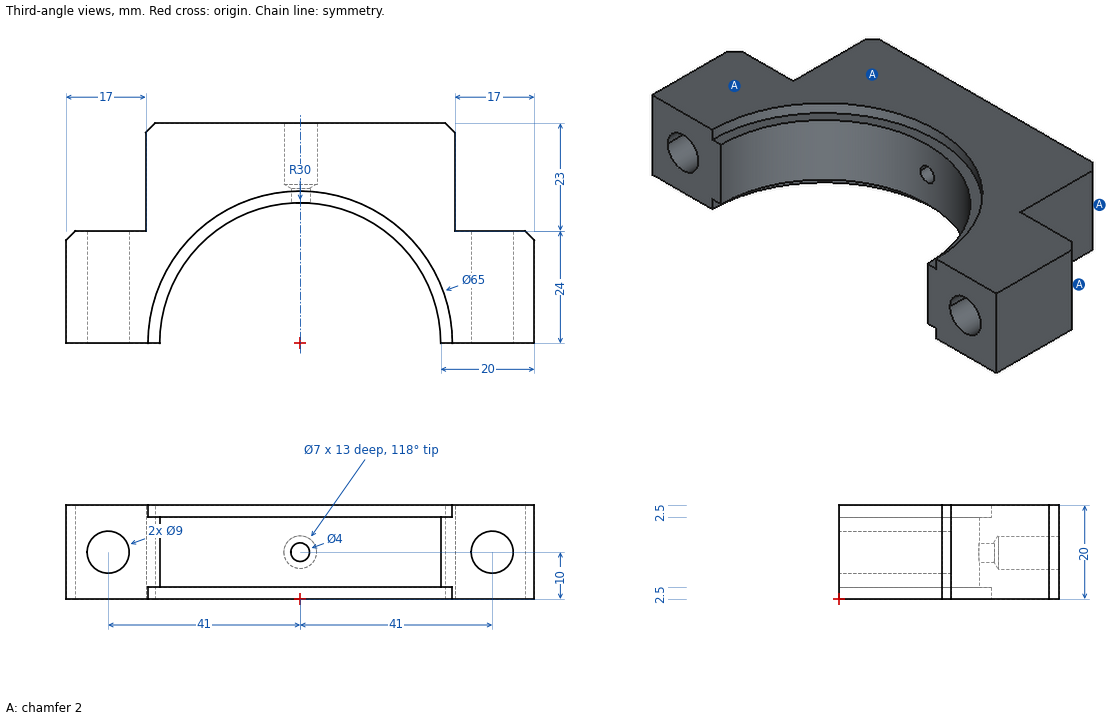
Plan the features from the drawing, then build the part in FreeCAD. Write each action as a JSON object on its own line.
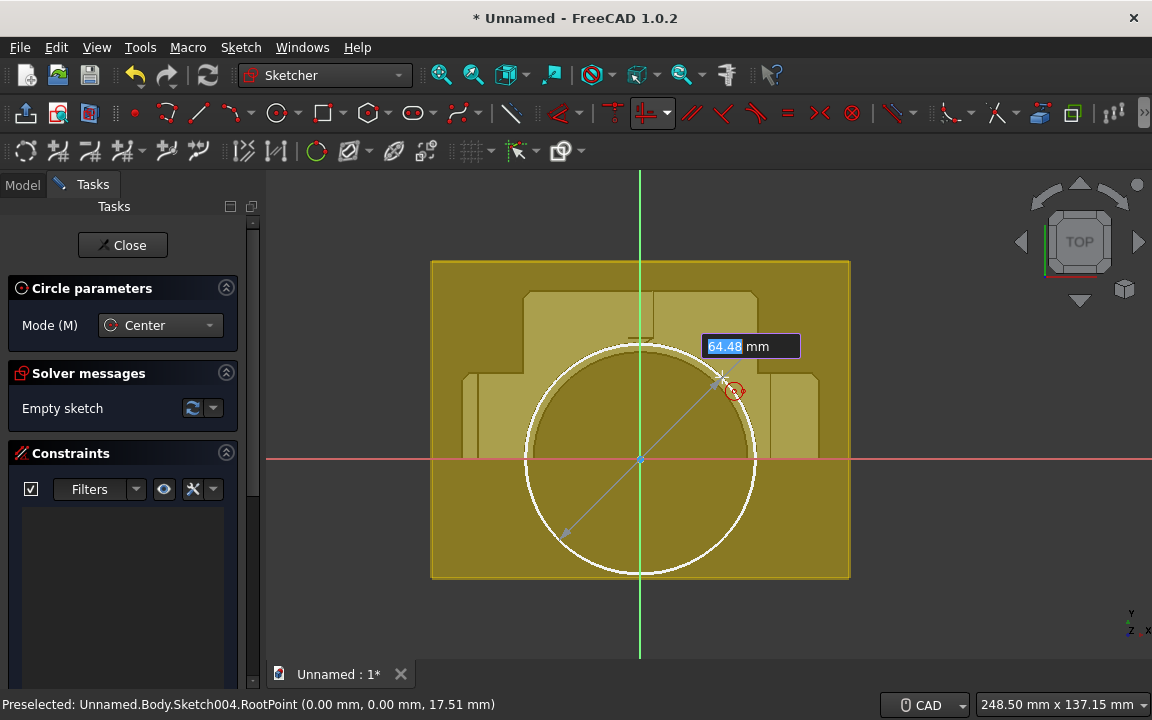
{"action": "type", "text": "65"}
{"action": "key", "text": "Return"}
{"action": "key", "text": "Escape"}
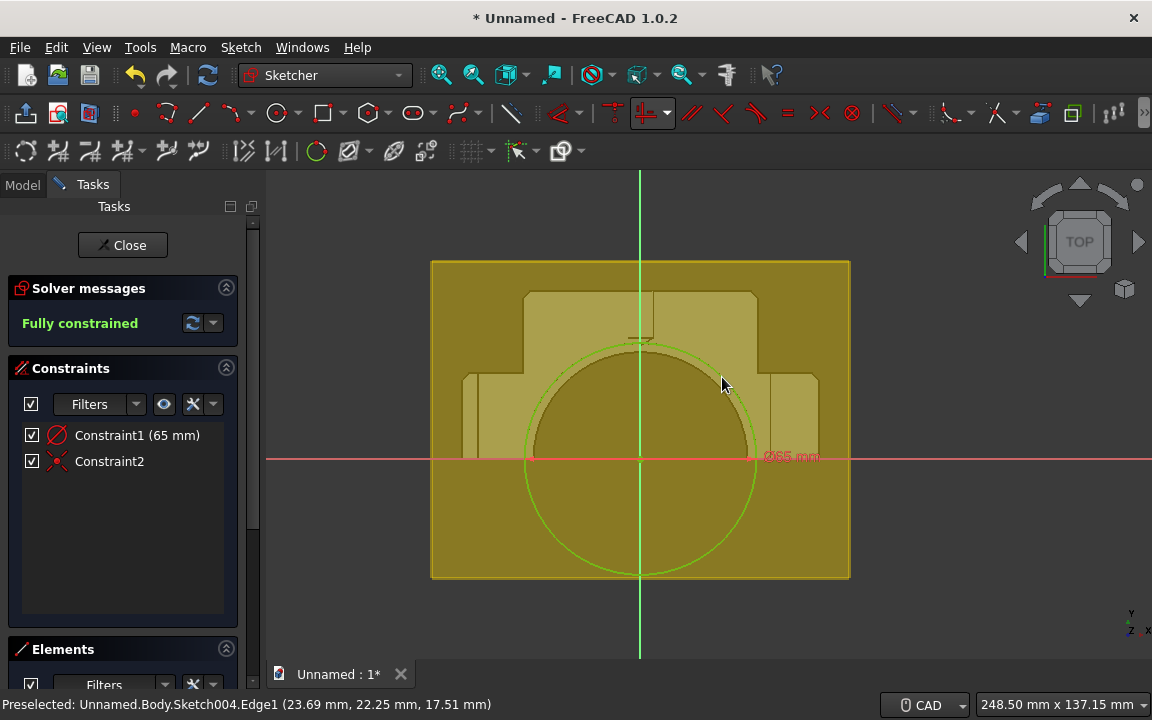
{"action": "left_click", "coordinate": [123, 245]}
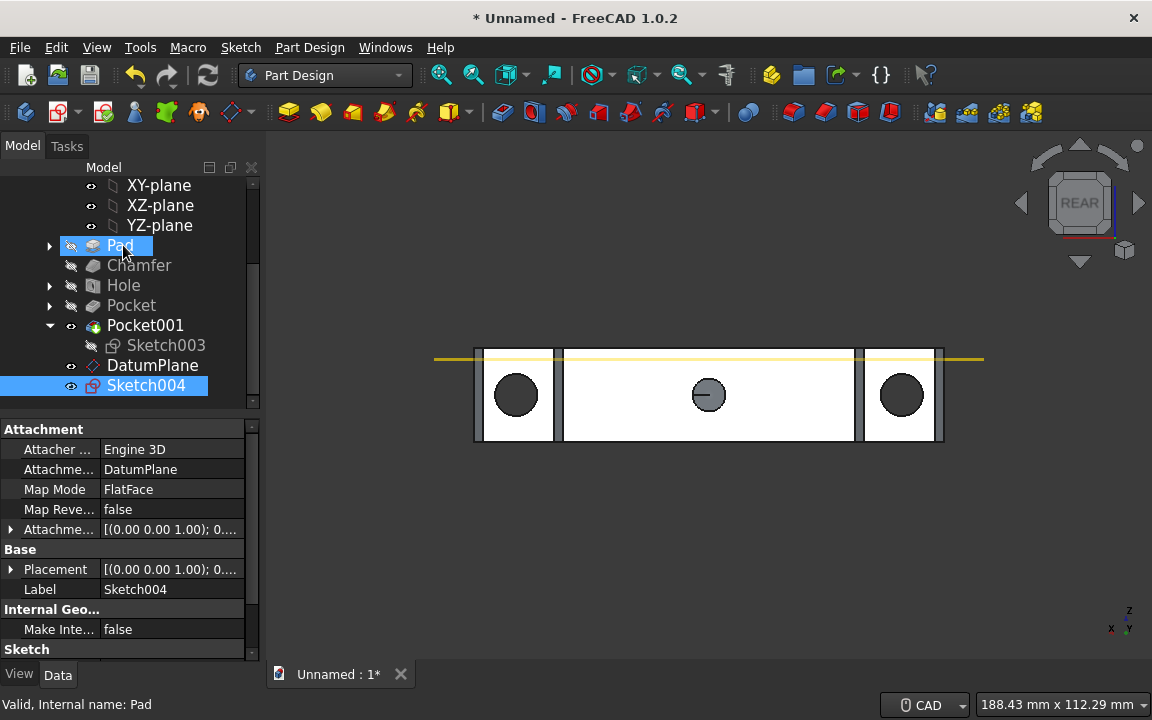
{"action": "left_click", "coordinate": [504, 112]}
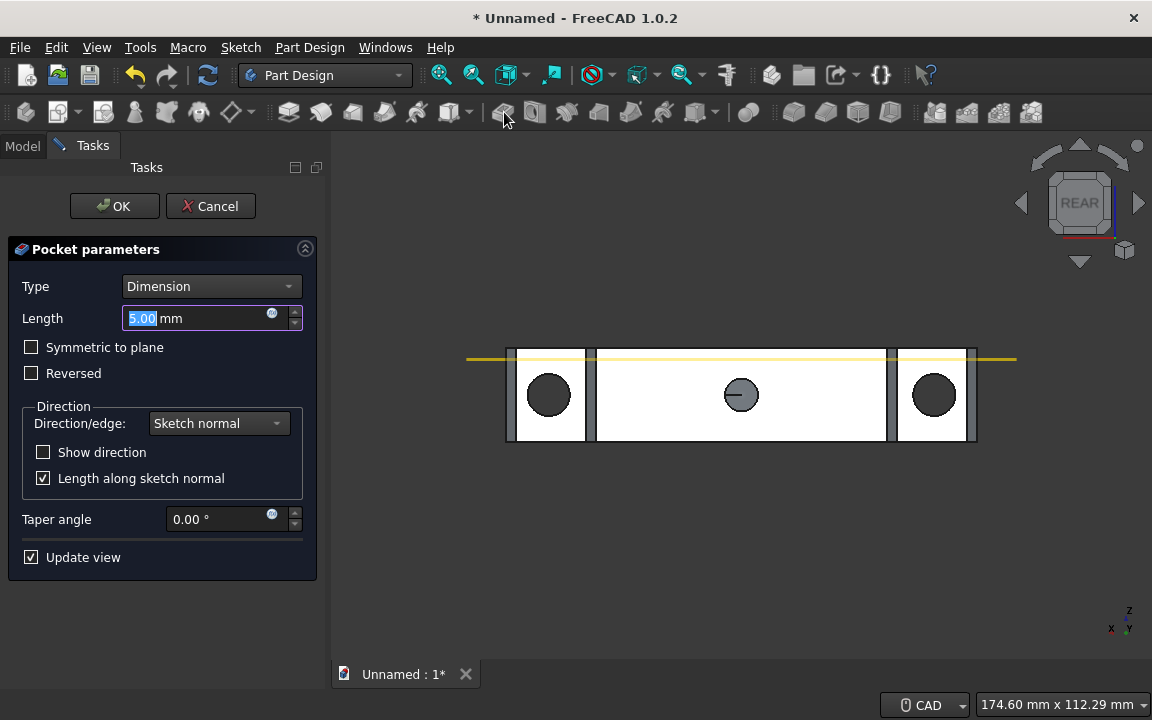
{"action": "type", "text": "2.5"}
{"action": "key", "text": "Tab"}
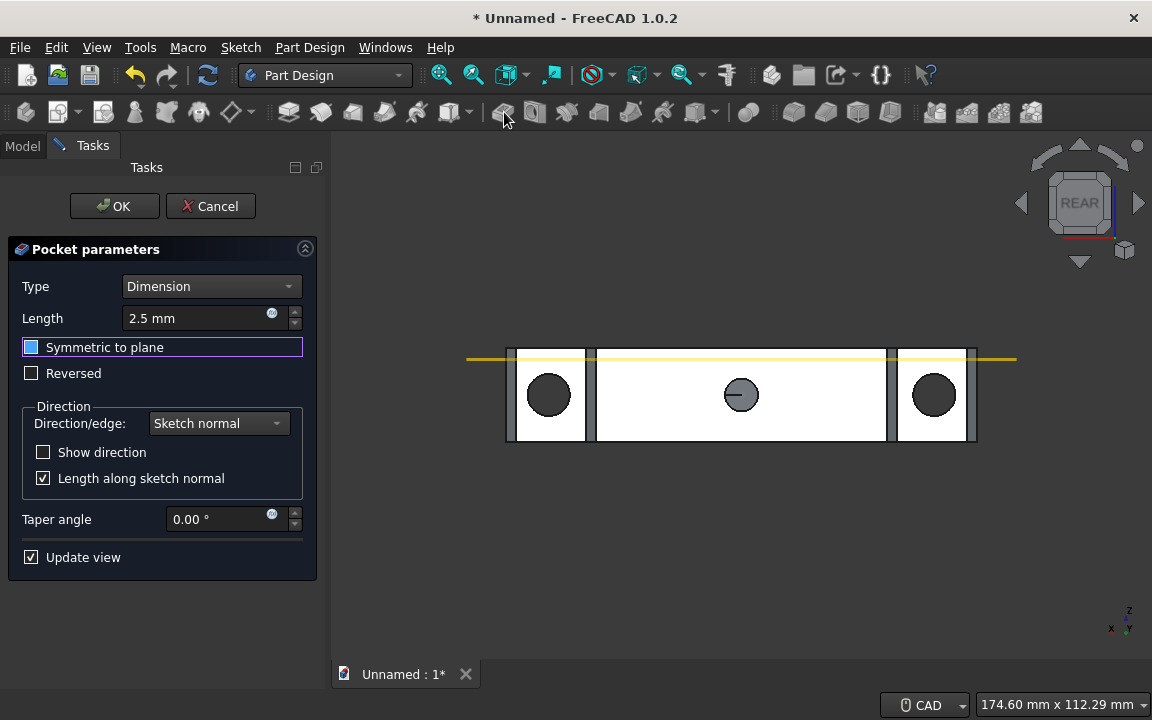
{"action": "left_click", "coordinate": [30, 373]}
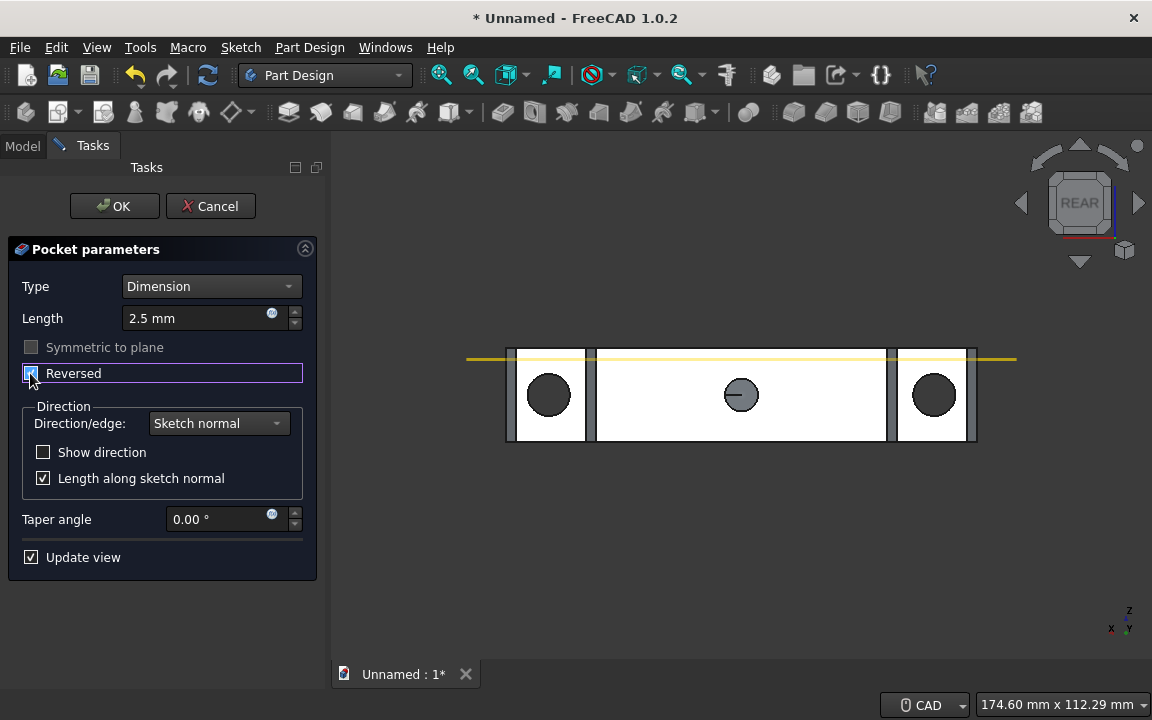
{"action": "left_click", "coordinate": [115, 206]}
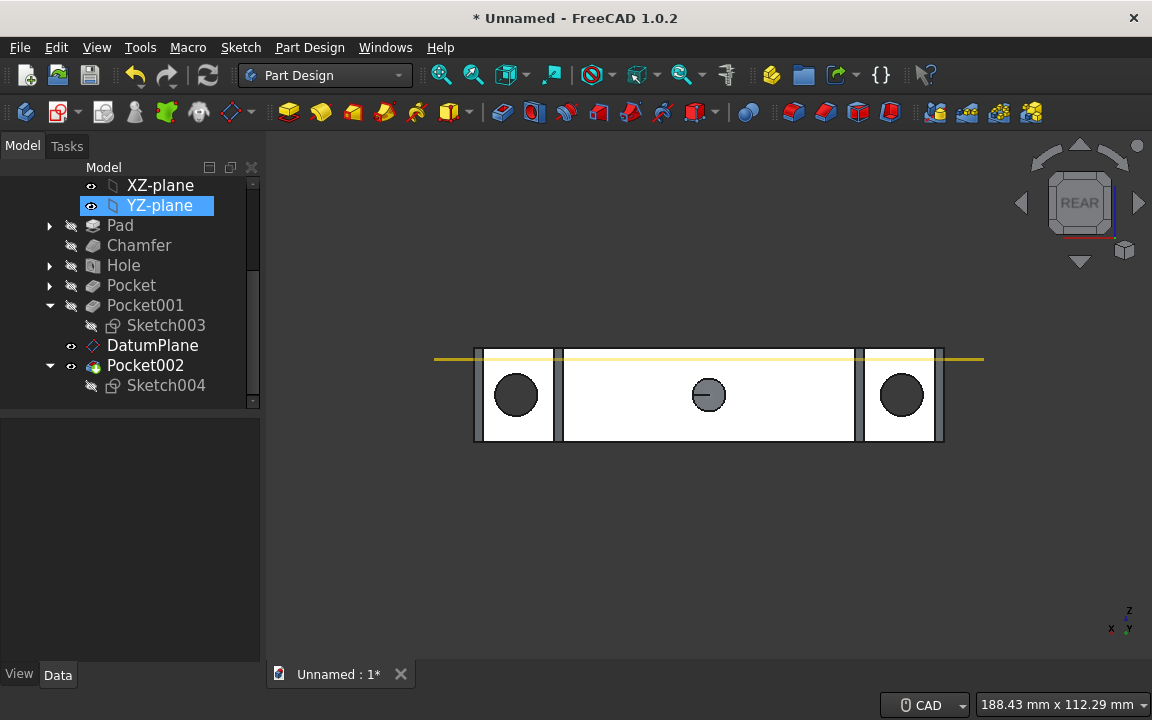
{"action": "left_click", "coordinate": [116, 346]}
{"action": "key", "text": "space"}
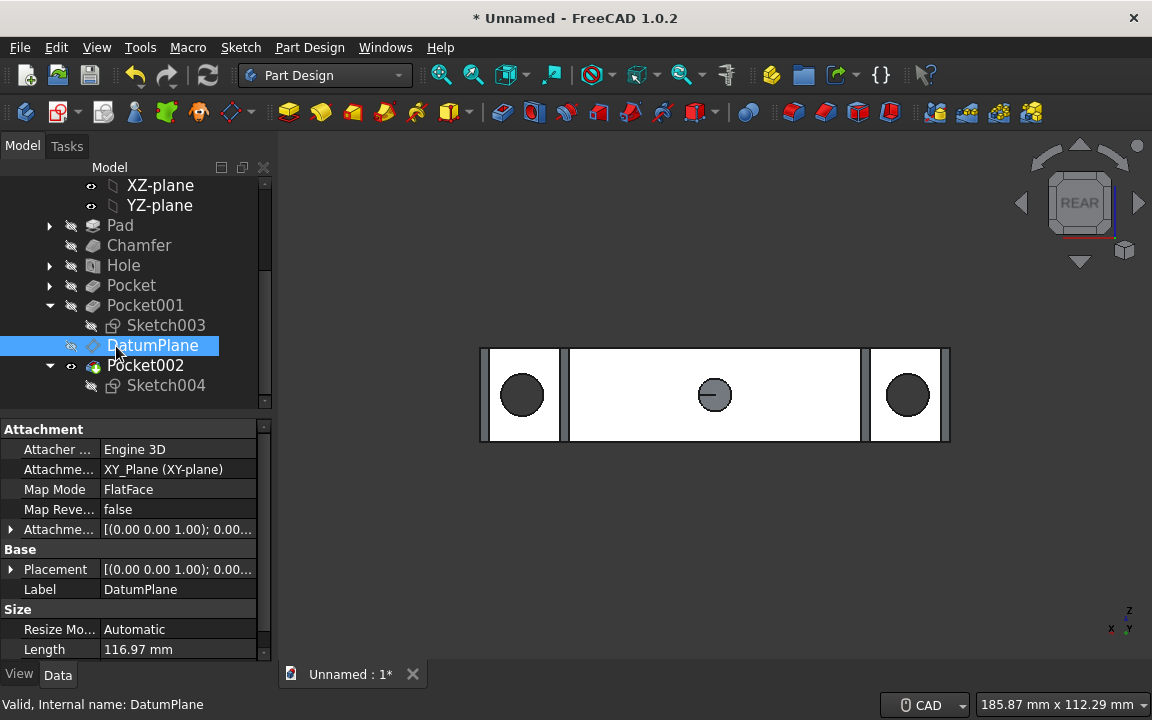
{"action": "left_click", "coordinate": [632, 394]}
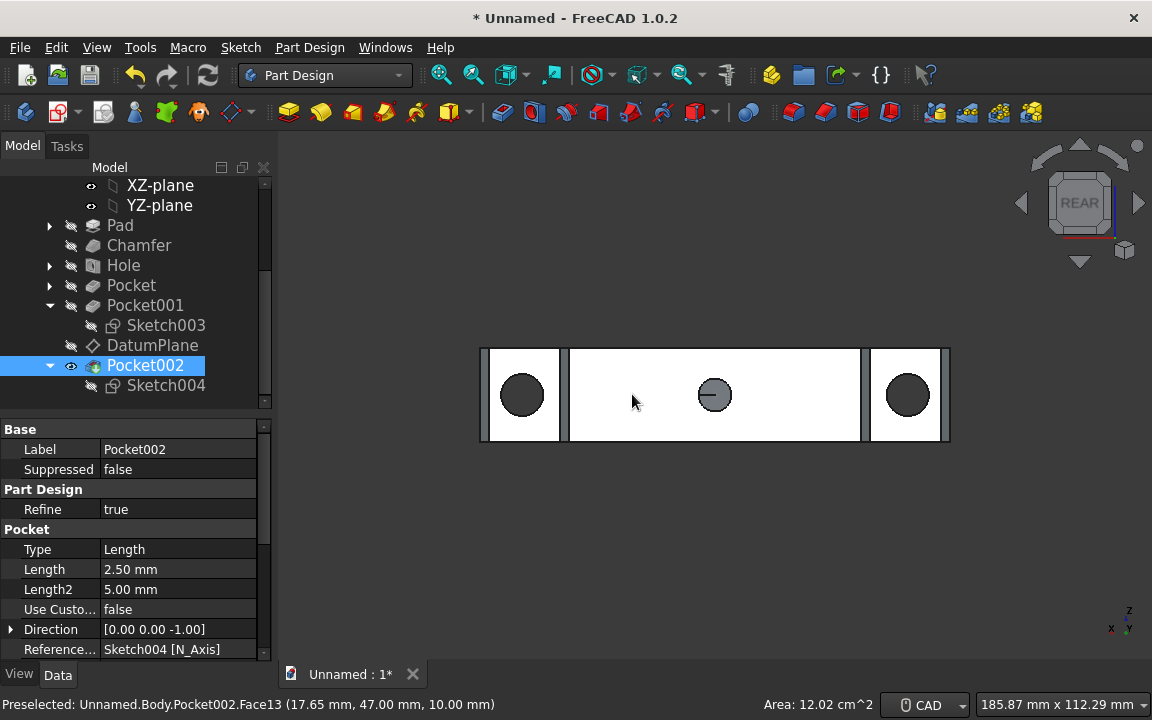
{"action": "left_click", "coordinate": [58, 112]}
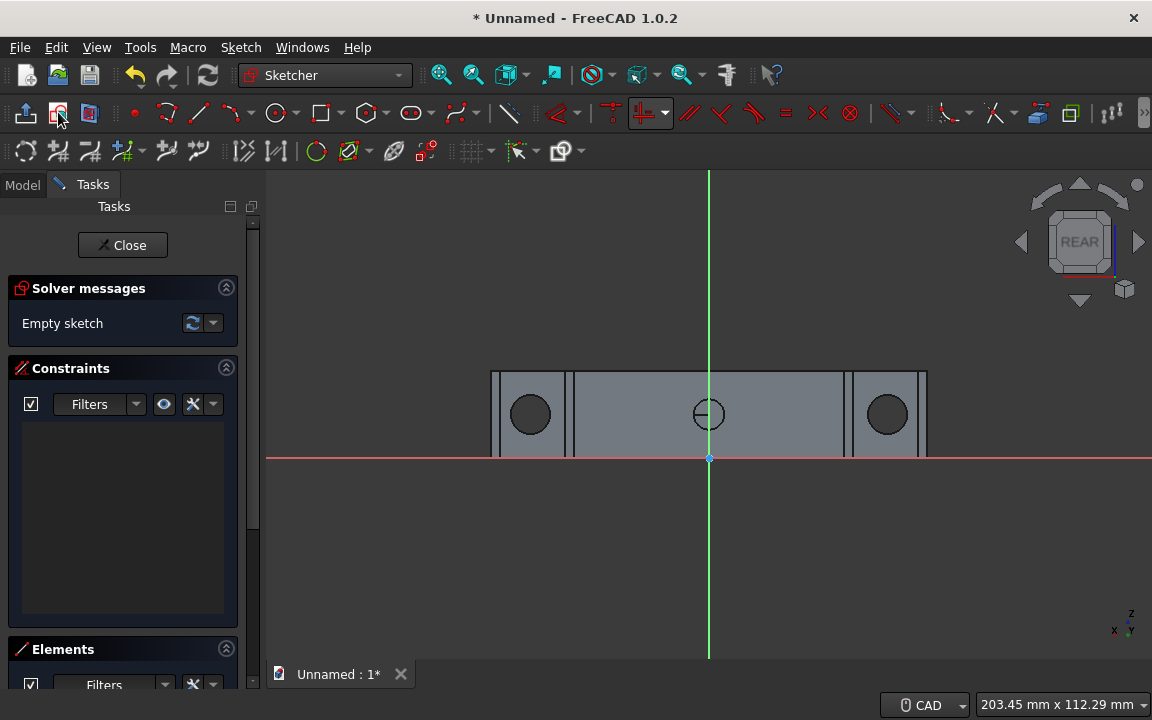
{"action": "scroll", "coordinate": [713, 415], "scroll_direction": "up", "scroll_amount": 14}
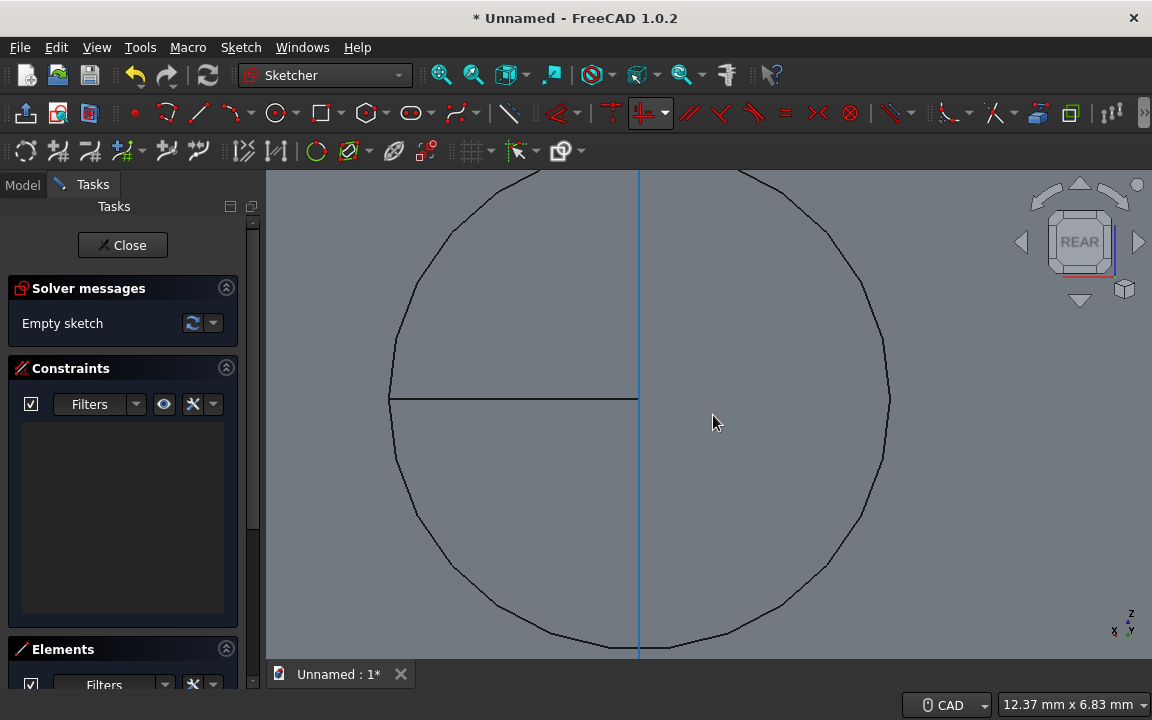
{"action": "left_click", "coordinate": [276, 114]}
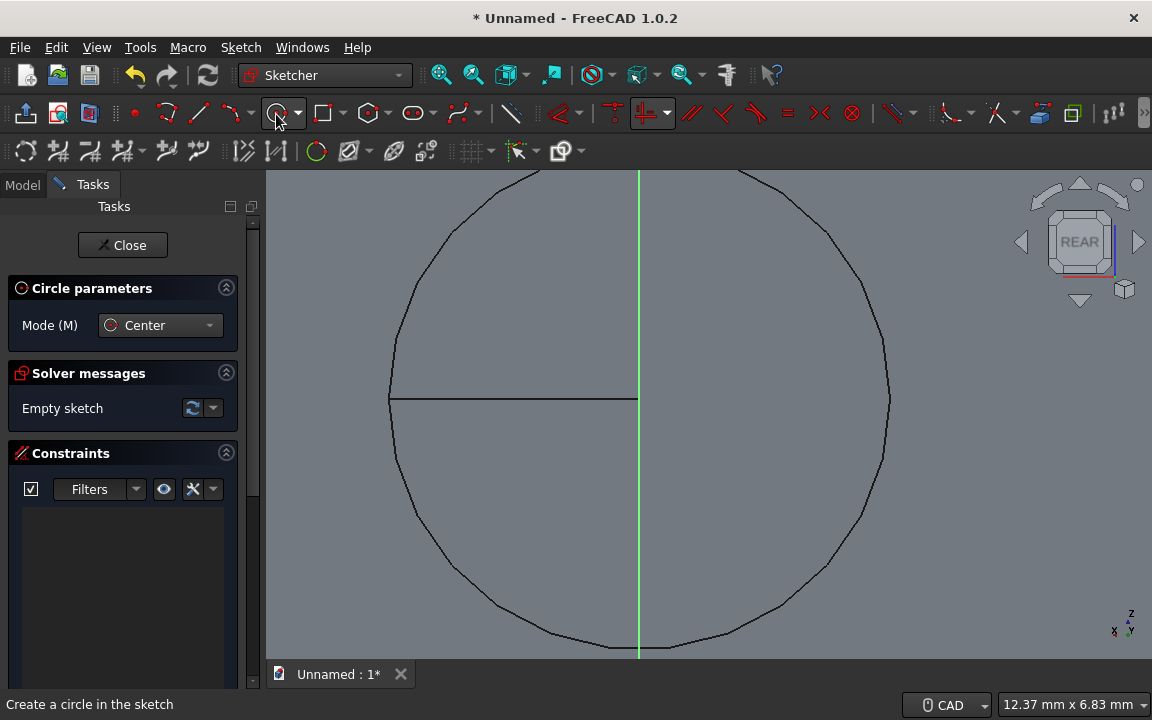
{"action": "left_click", "coordinate": [639, 399]}
{"action": "mouse_move", "coordinate": [741, 298]}